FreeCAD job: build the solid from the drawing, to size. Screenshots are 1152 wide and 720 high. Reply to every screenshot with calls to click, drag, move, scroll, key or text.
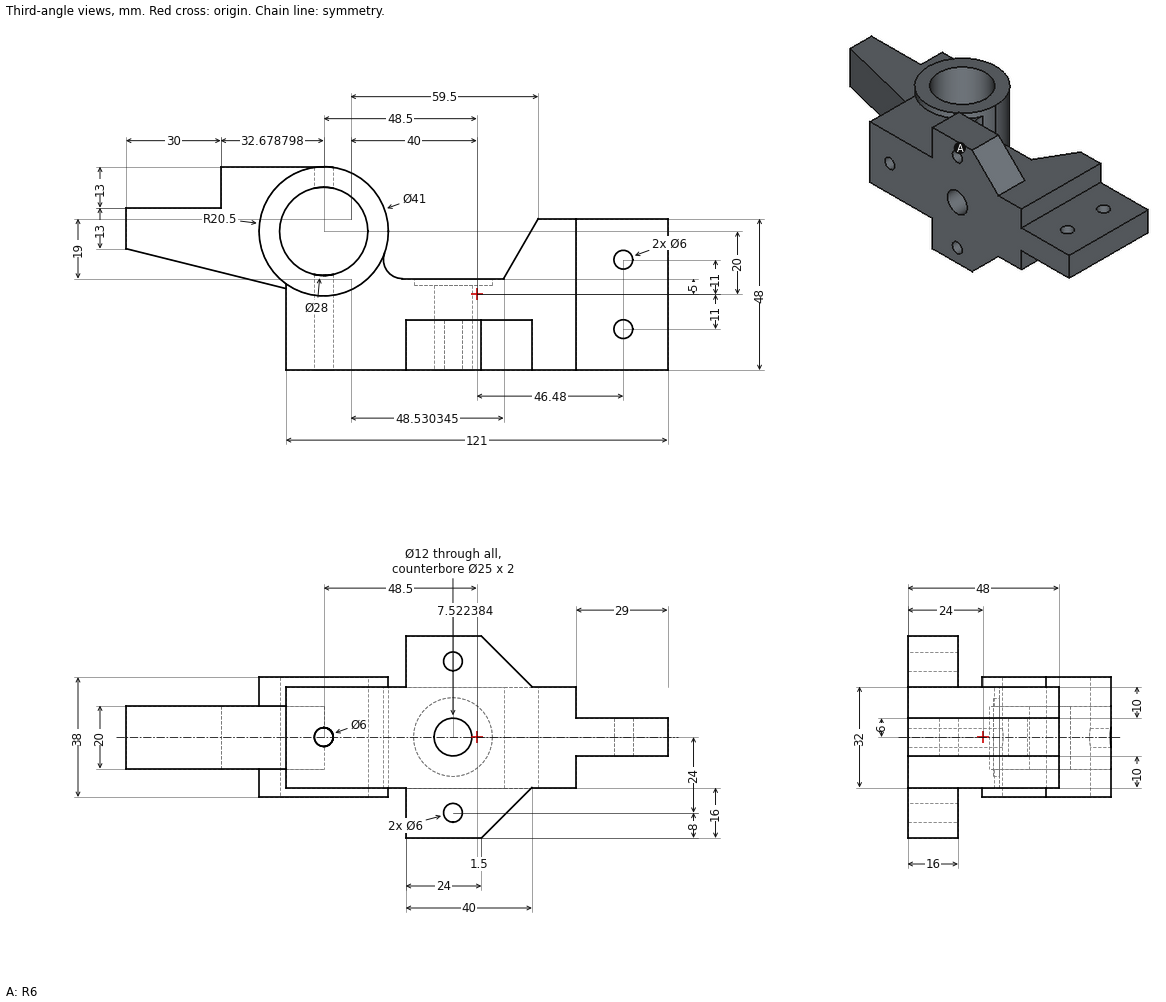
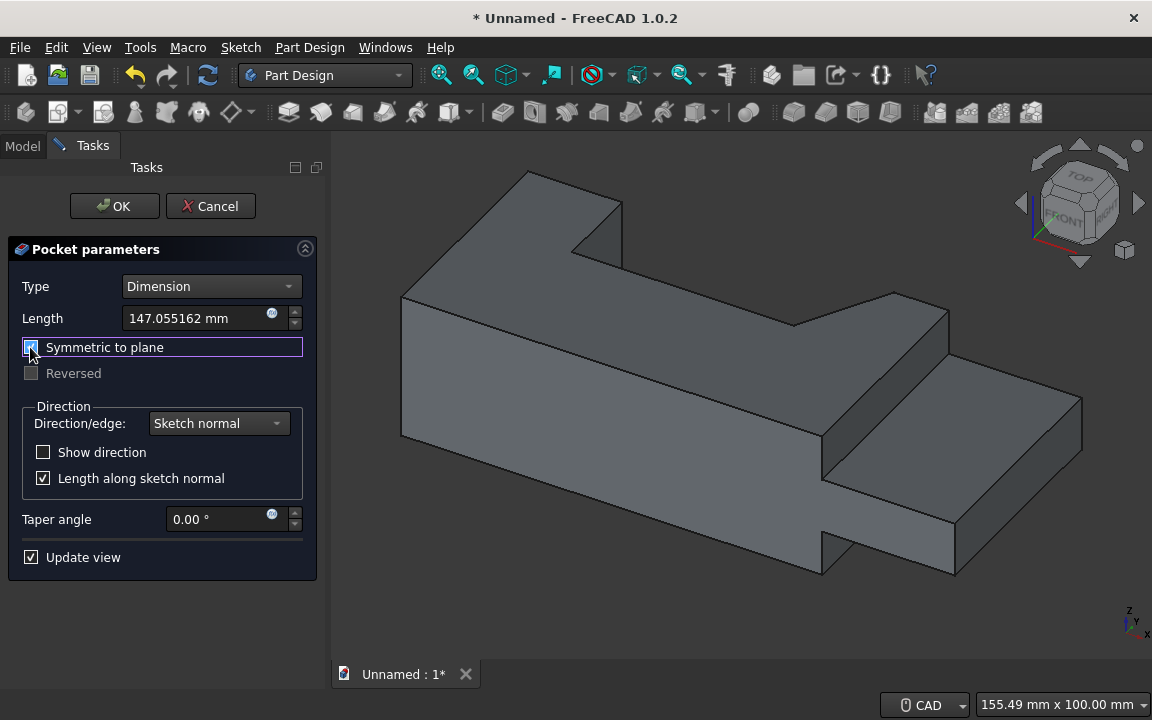
click(115, 206)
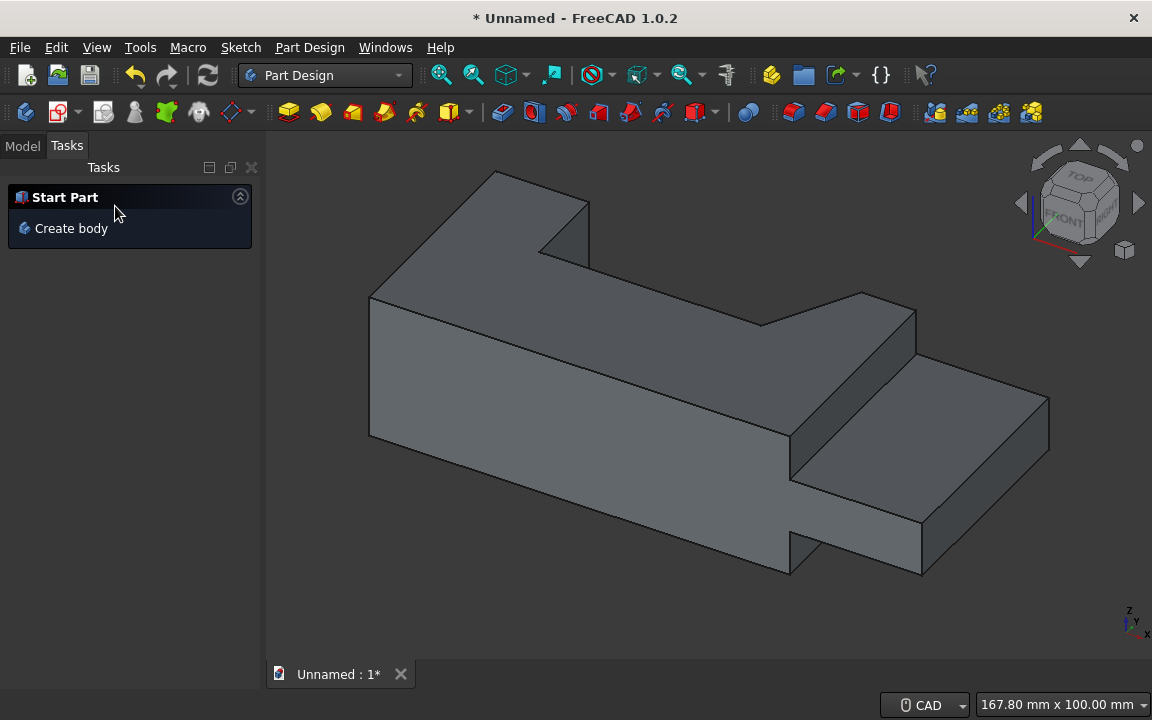
click(58, 112)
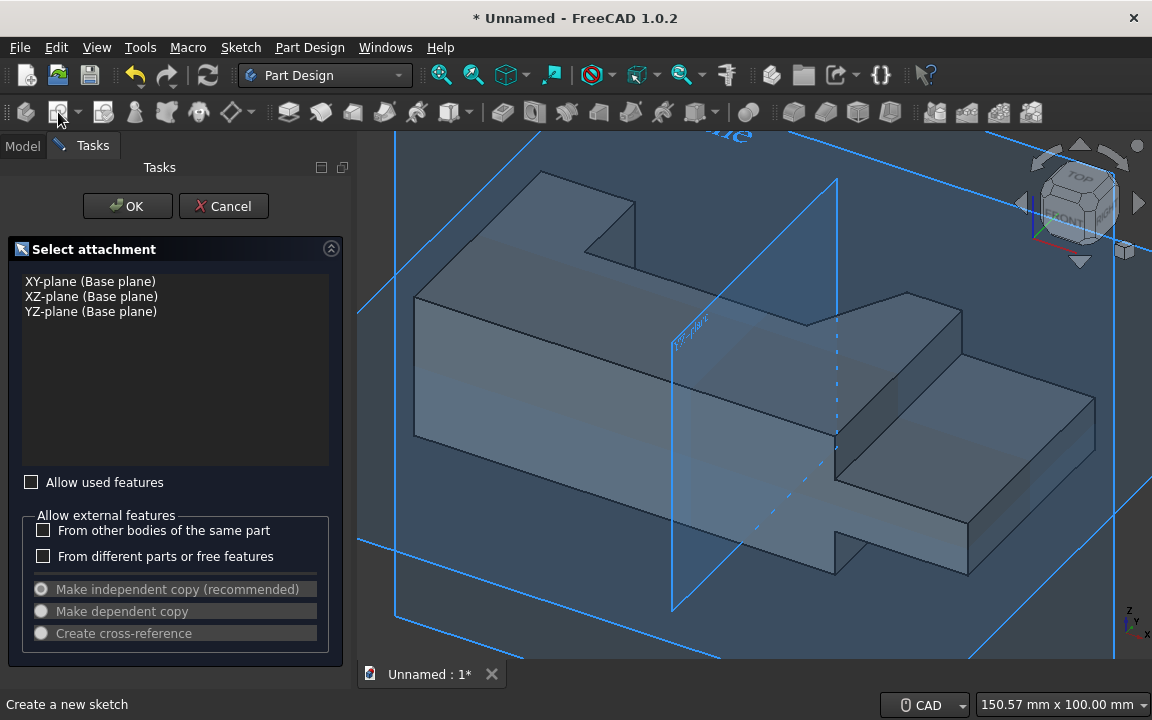
click(82, 282)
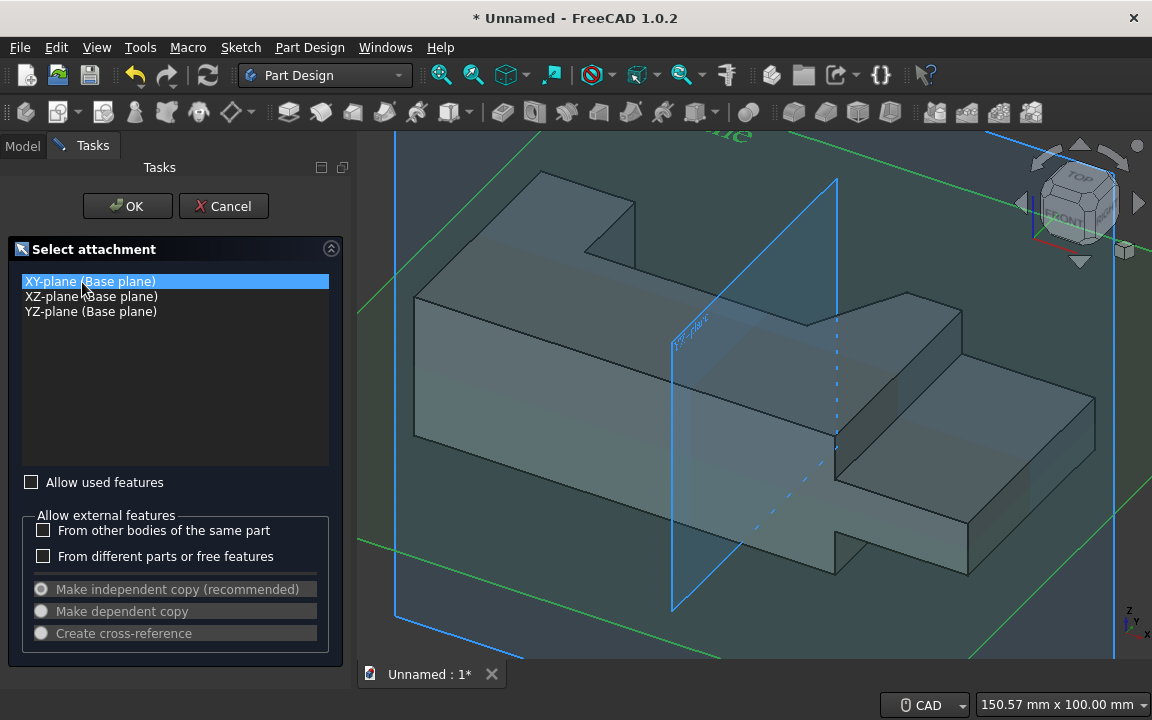
click(128, 206)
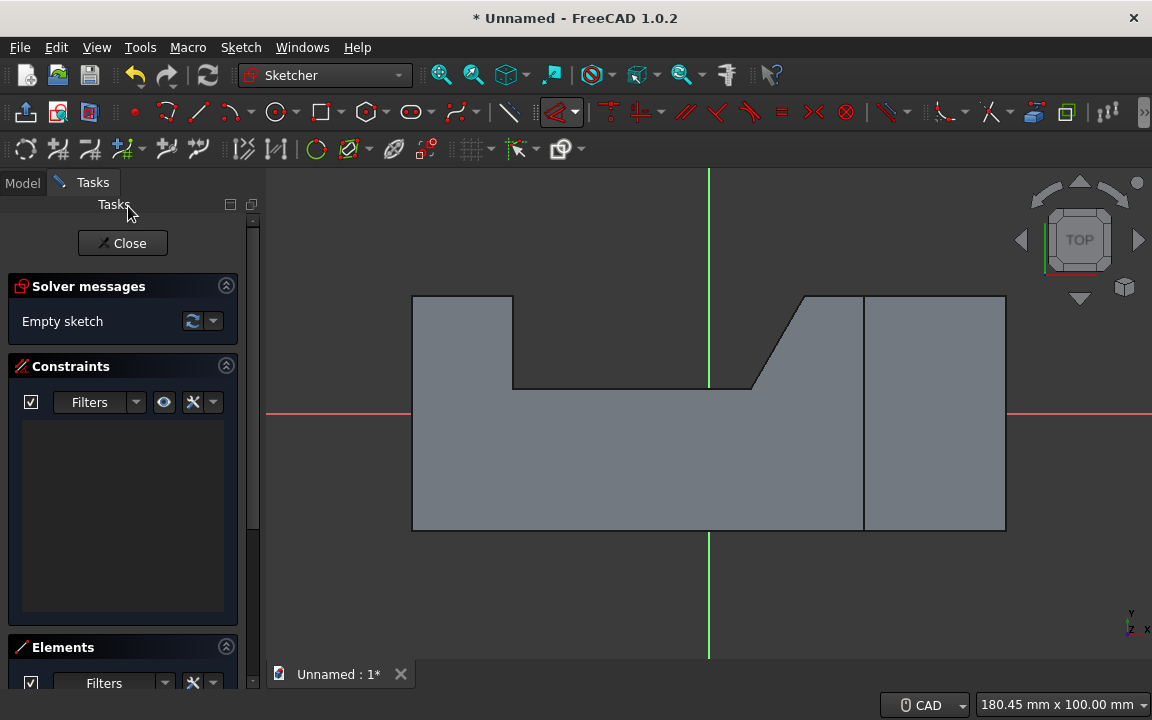
key(q)
key(s)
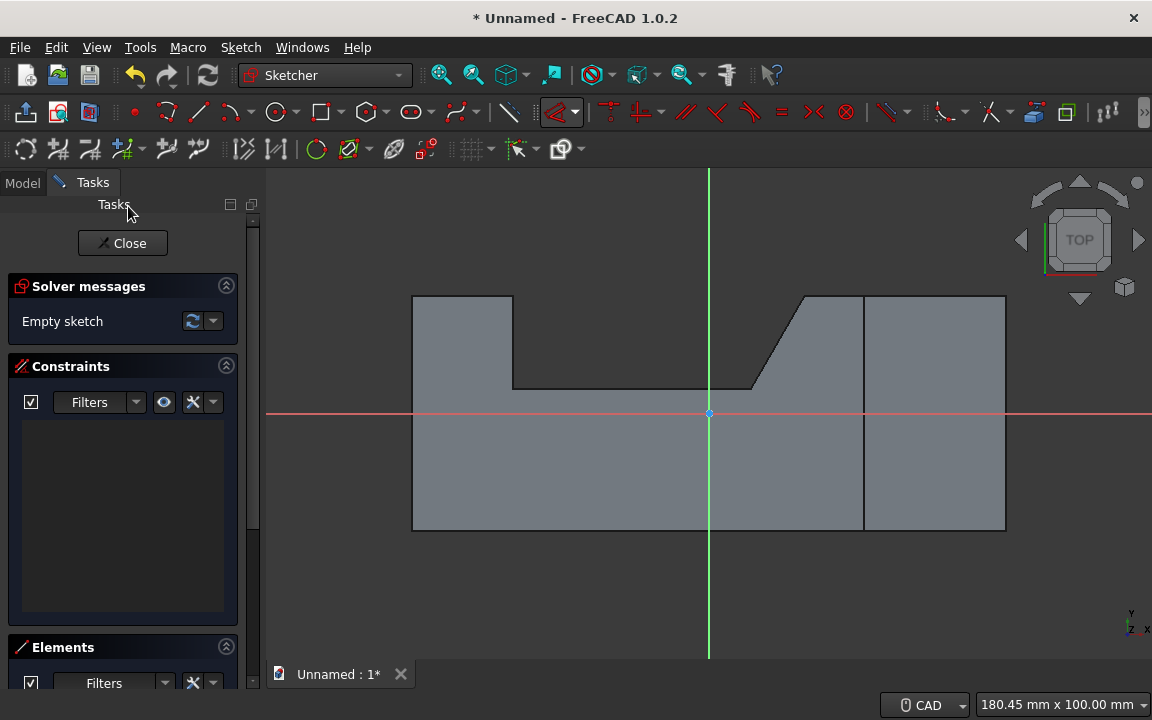
scroll(334, 196, up, 2)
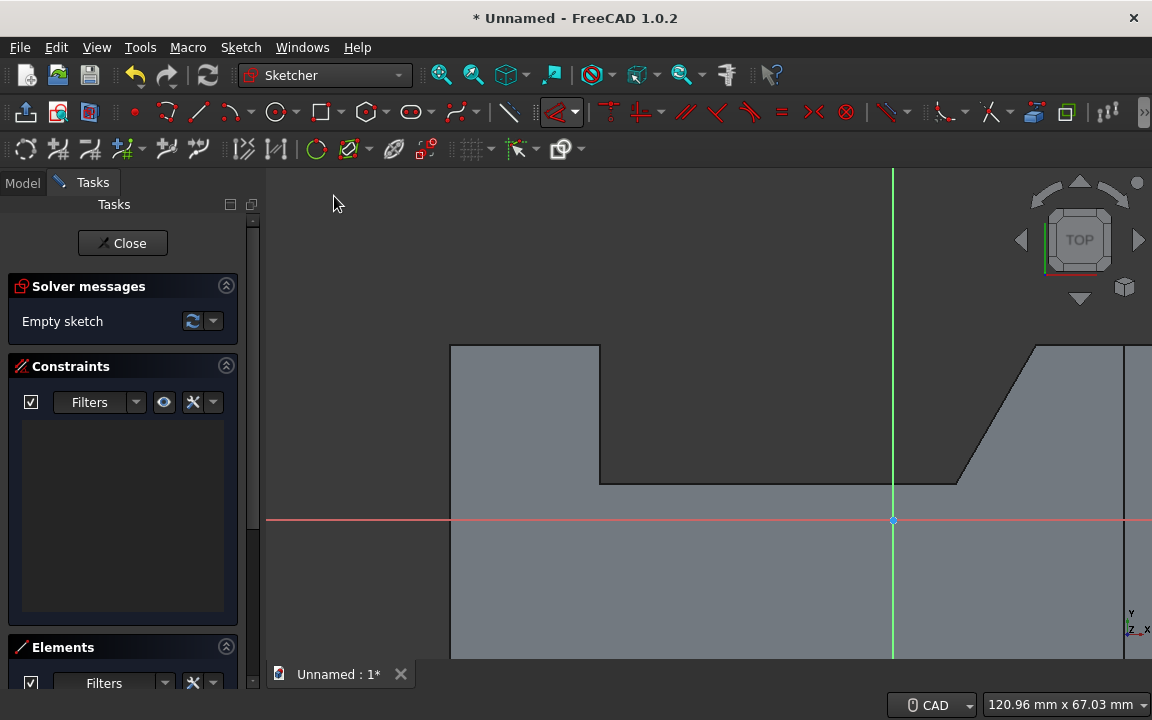
key(g)
key(c)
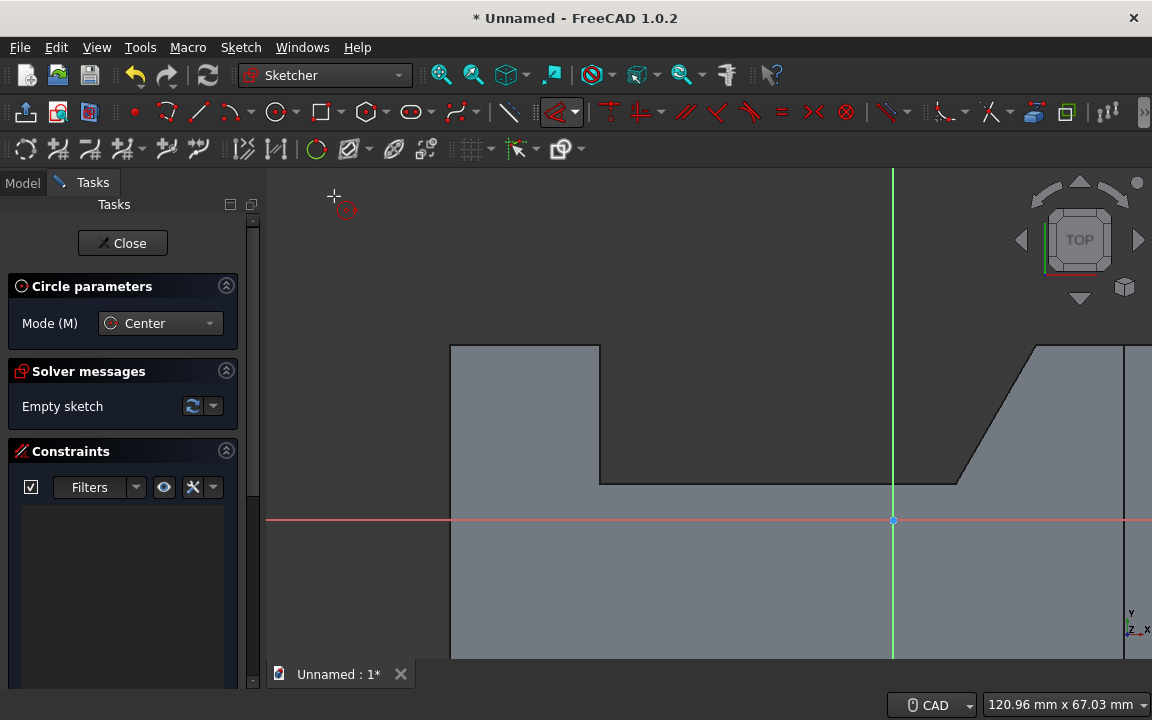
click(538, 374)
move(644, 268)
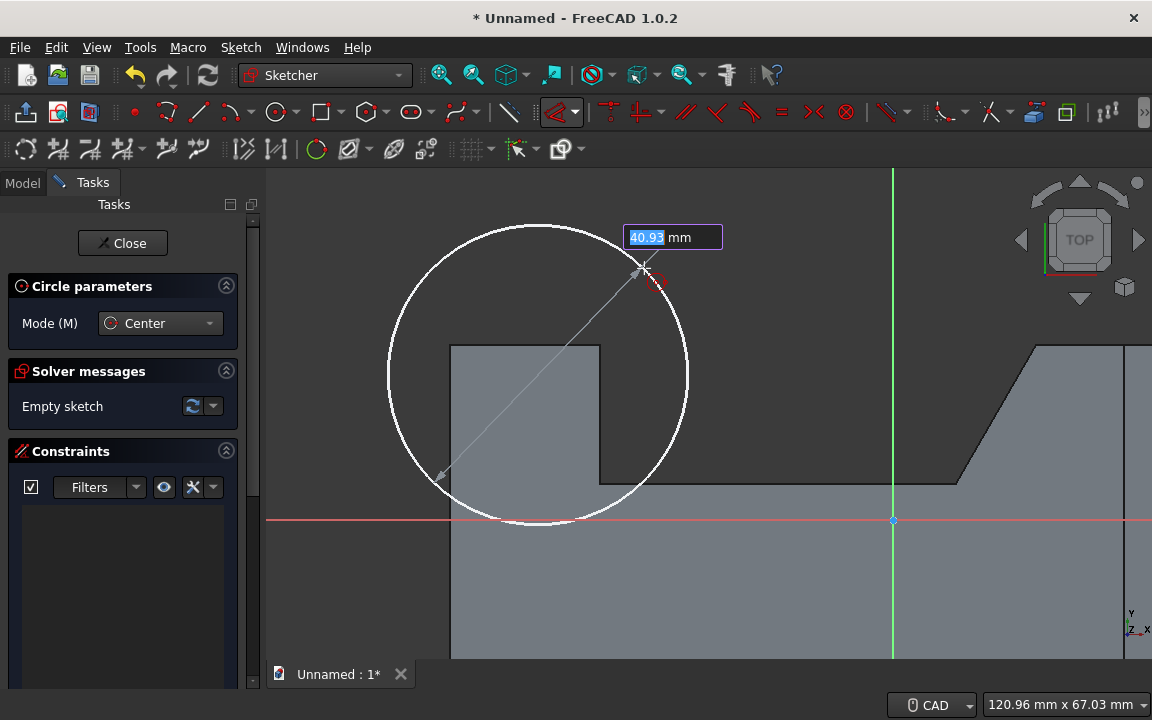
text(41)
key(Return)
key(Escape)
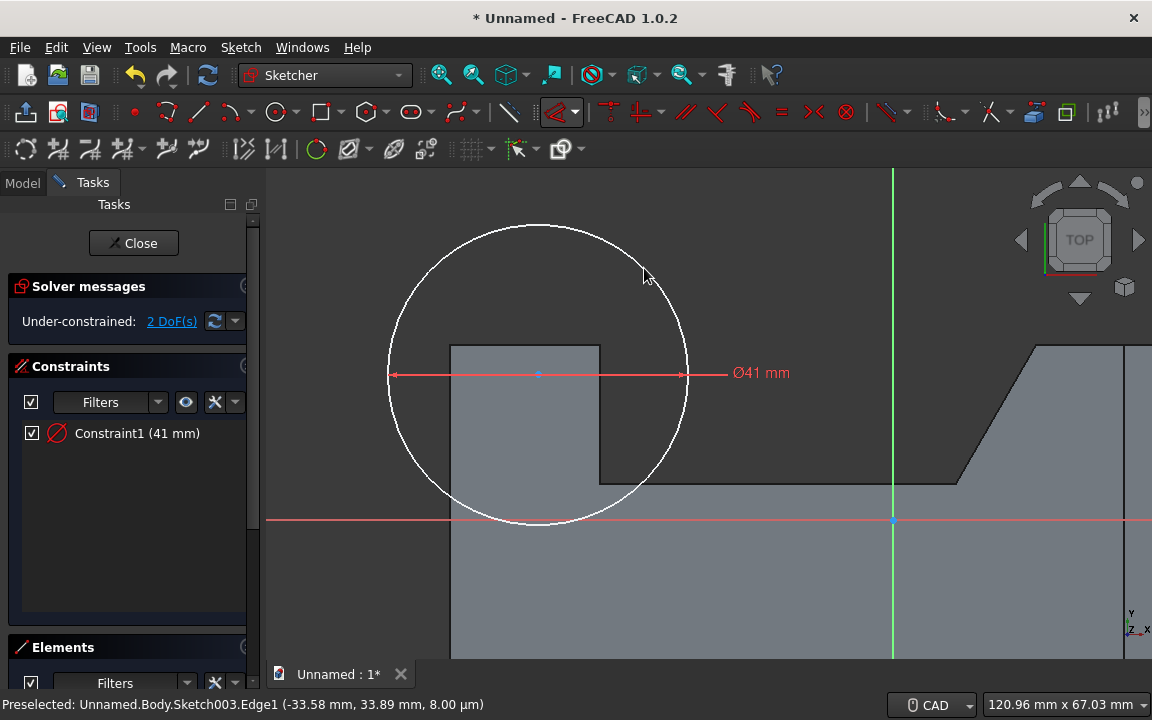
click(538, 375)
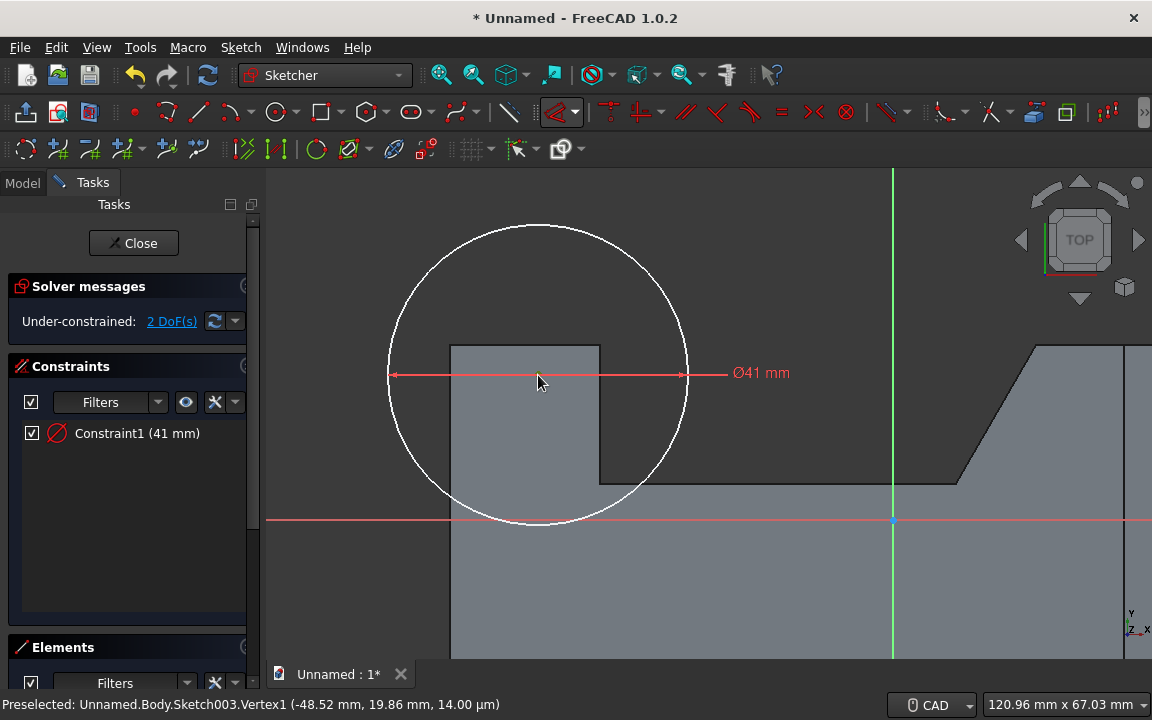
key(i)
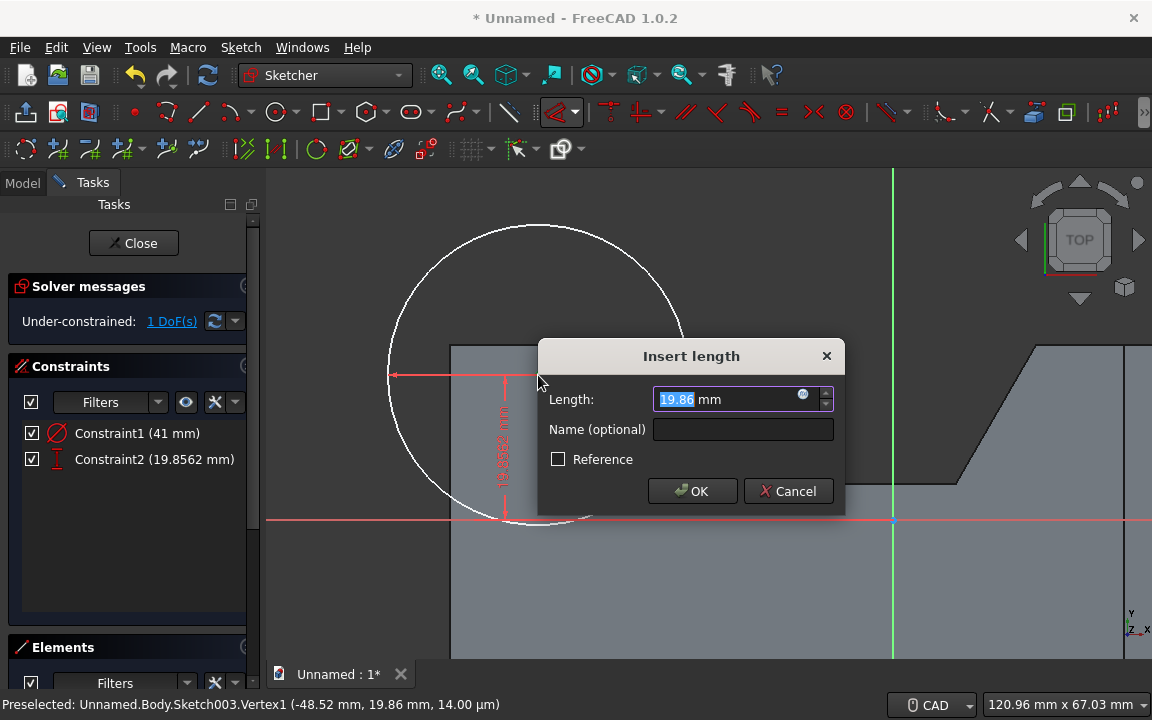
text(20)
key(Return)